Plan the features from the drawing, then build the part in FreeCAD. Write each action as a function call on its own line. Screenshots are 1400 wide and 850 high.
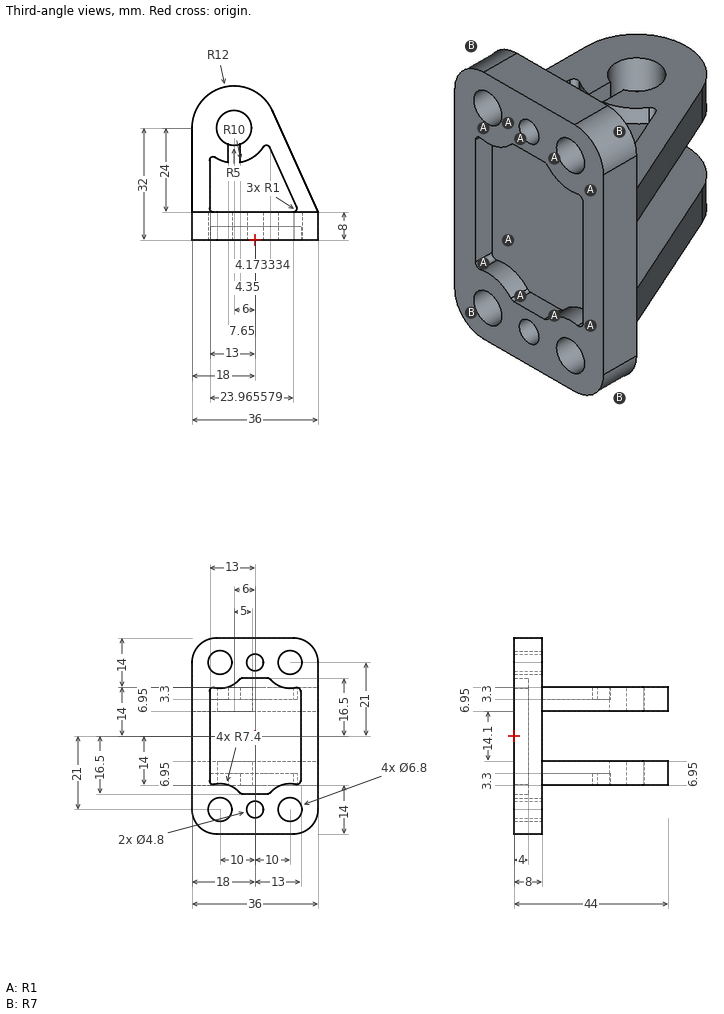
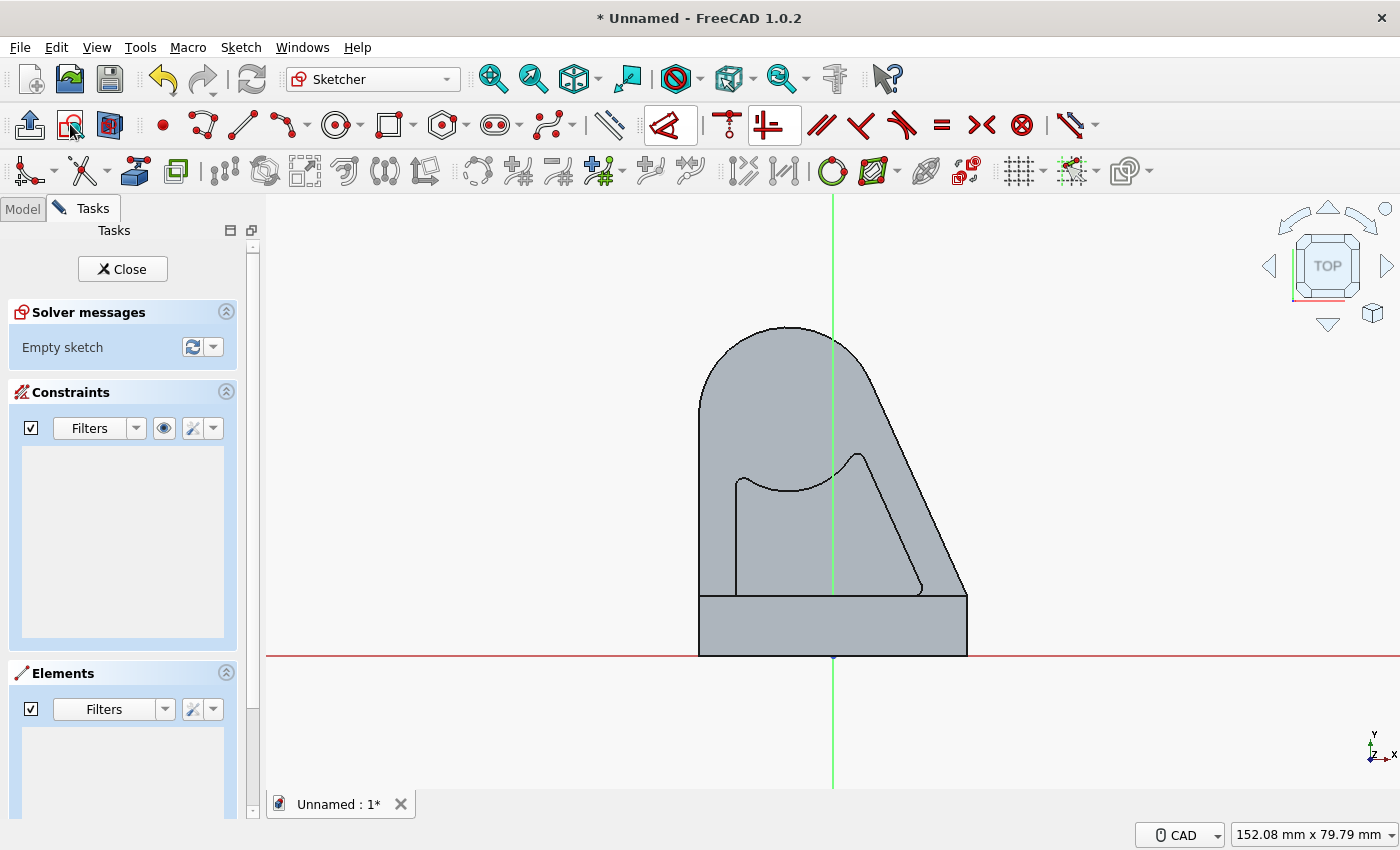
key(q)
key(s)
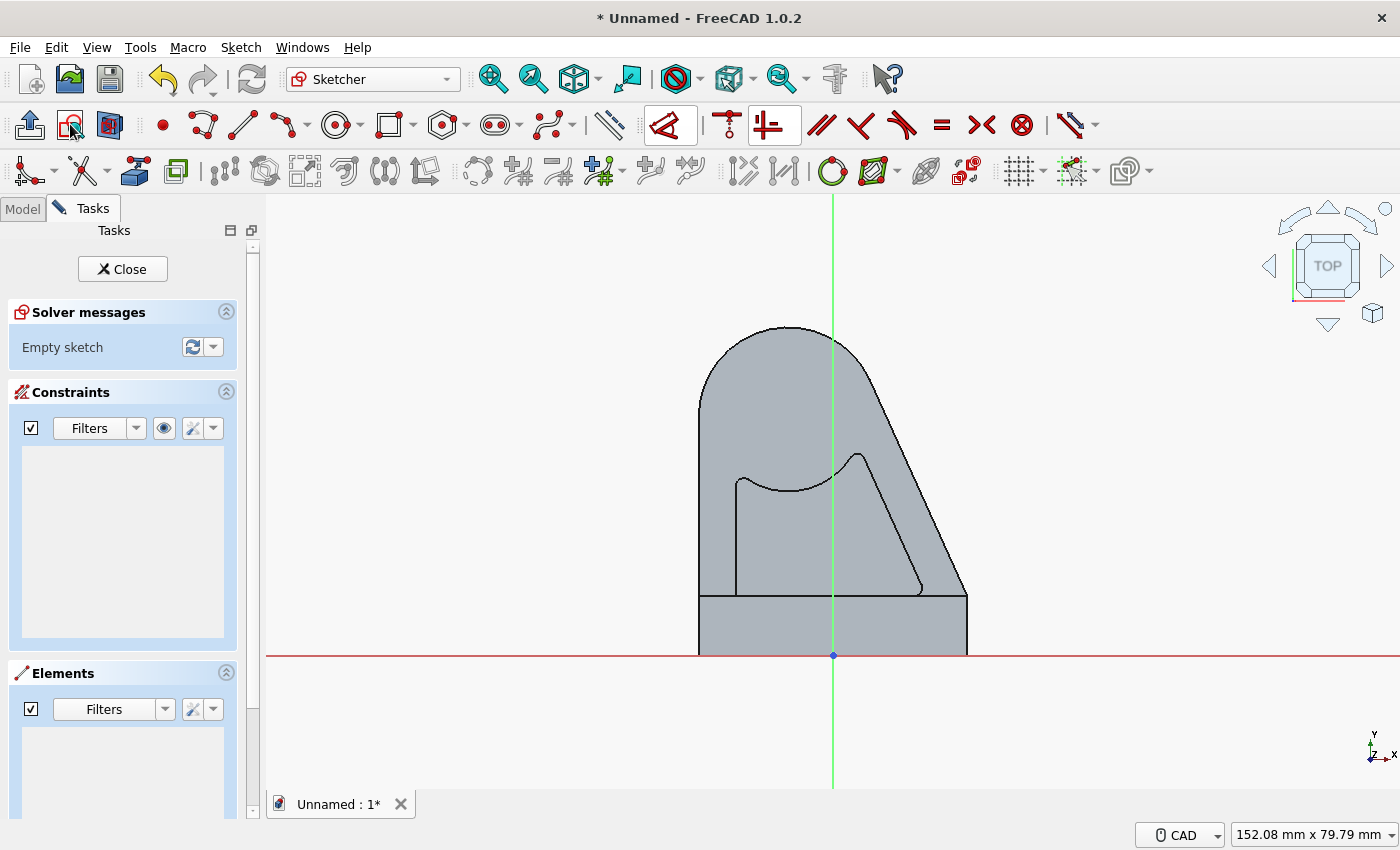
scroll(791, 469, up, 11)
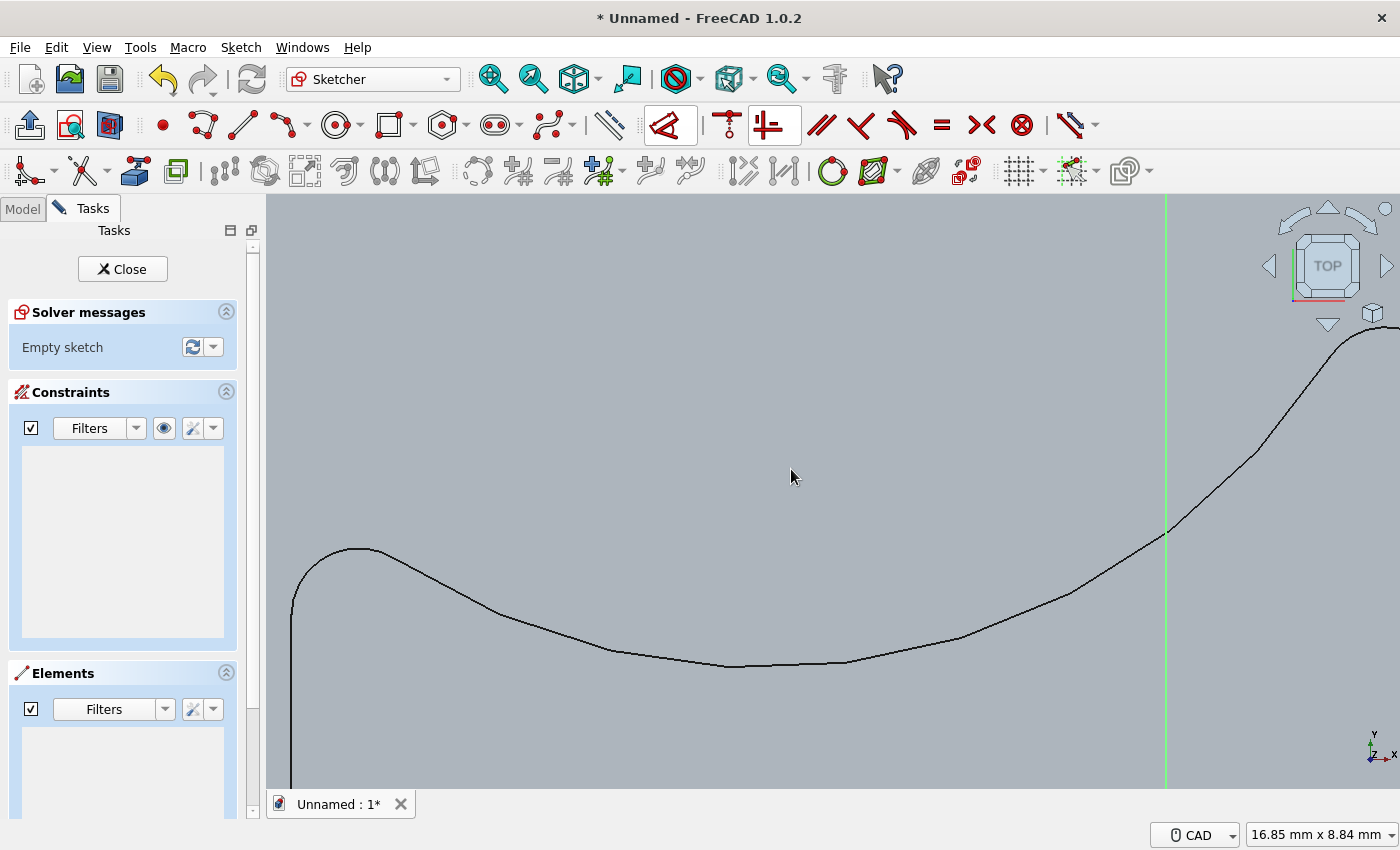
click(244, 126)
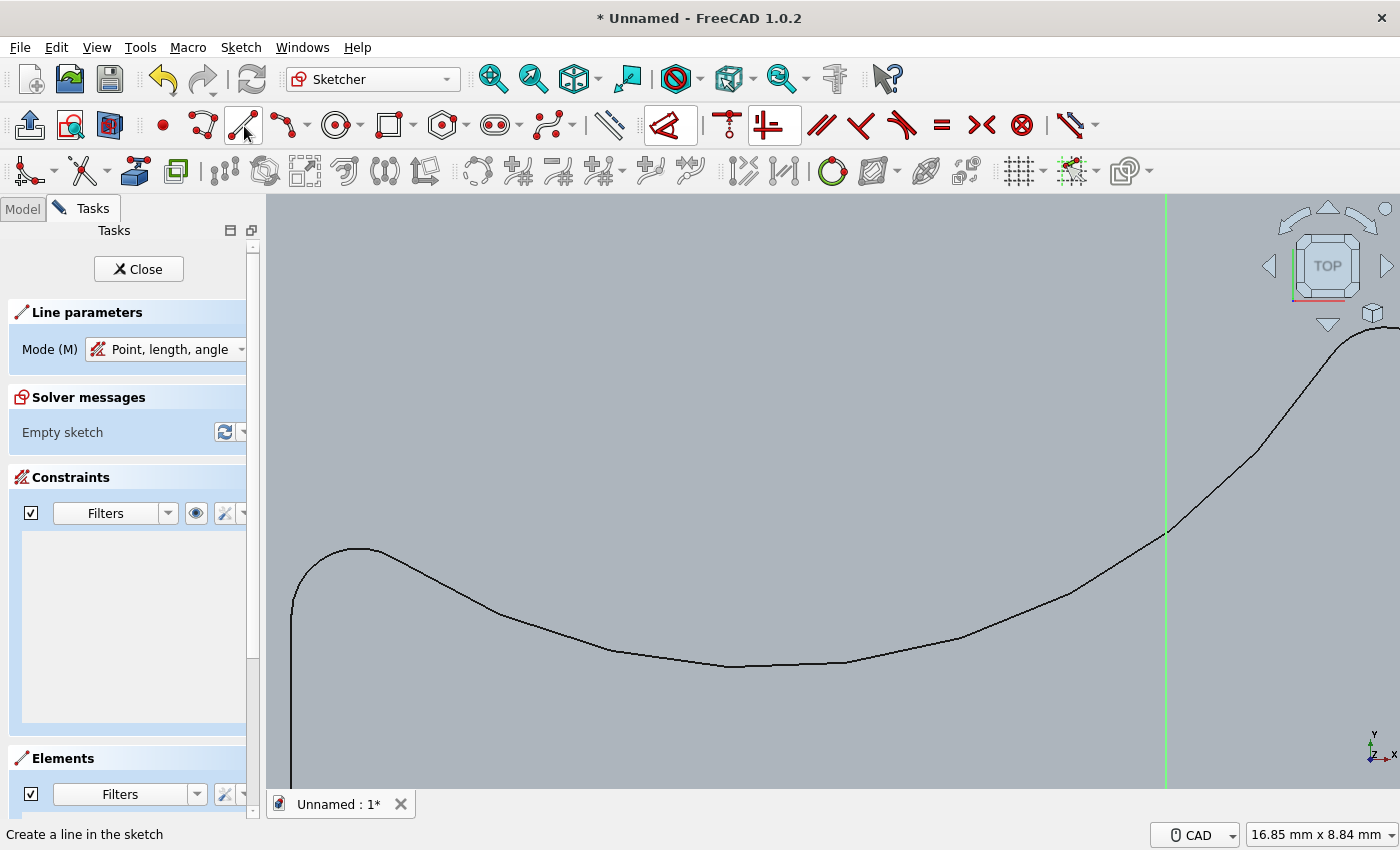
click(652, 313)
click(652, 659)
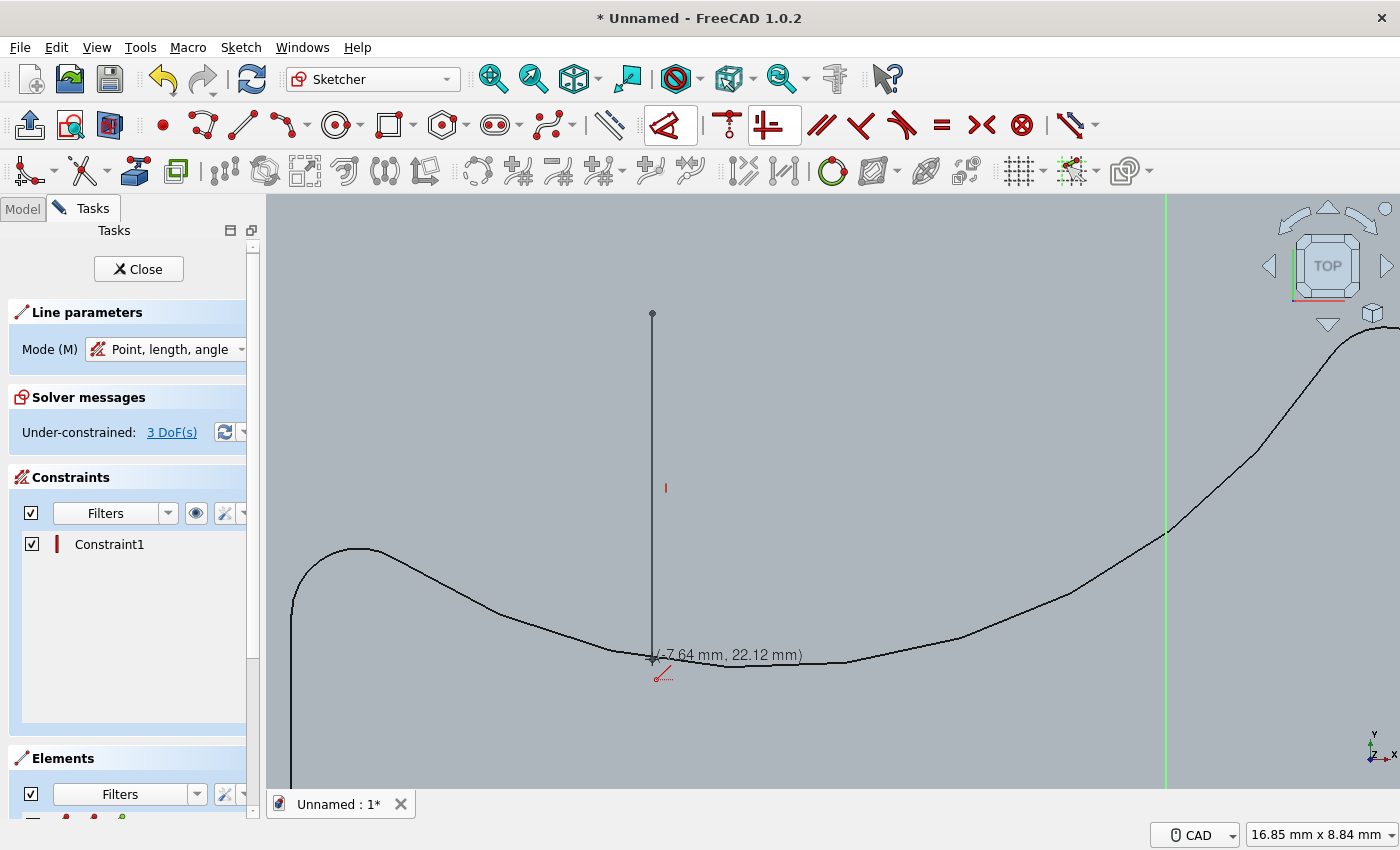
click(874, 659)
click(874, 313)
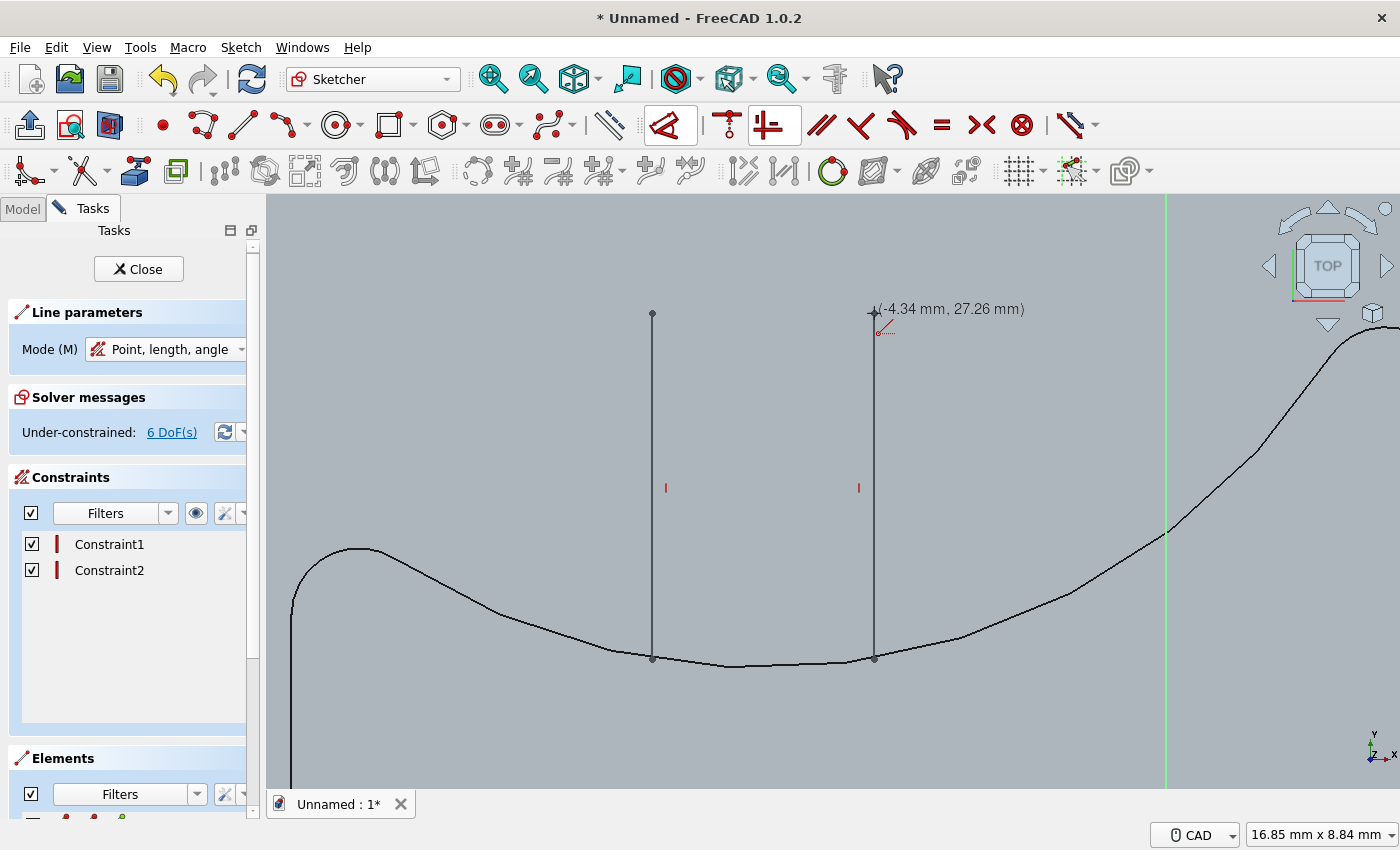
click(284, 126)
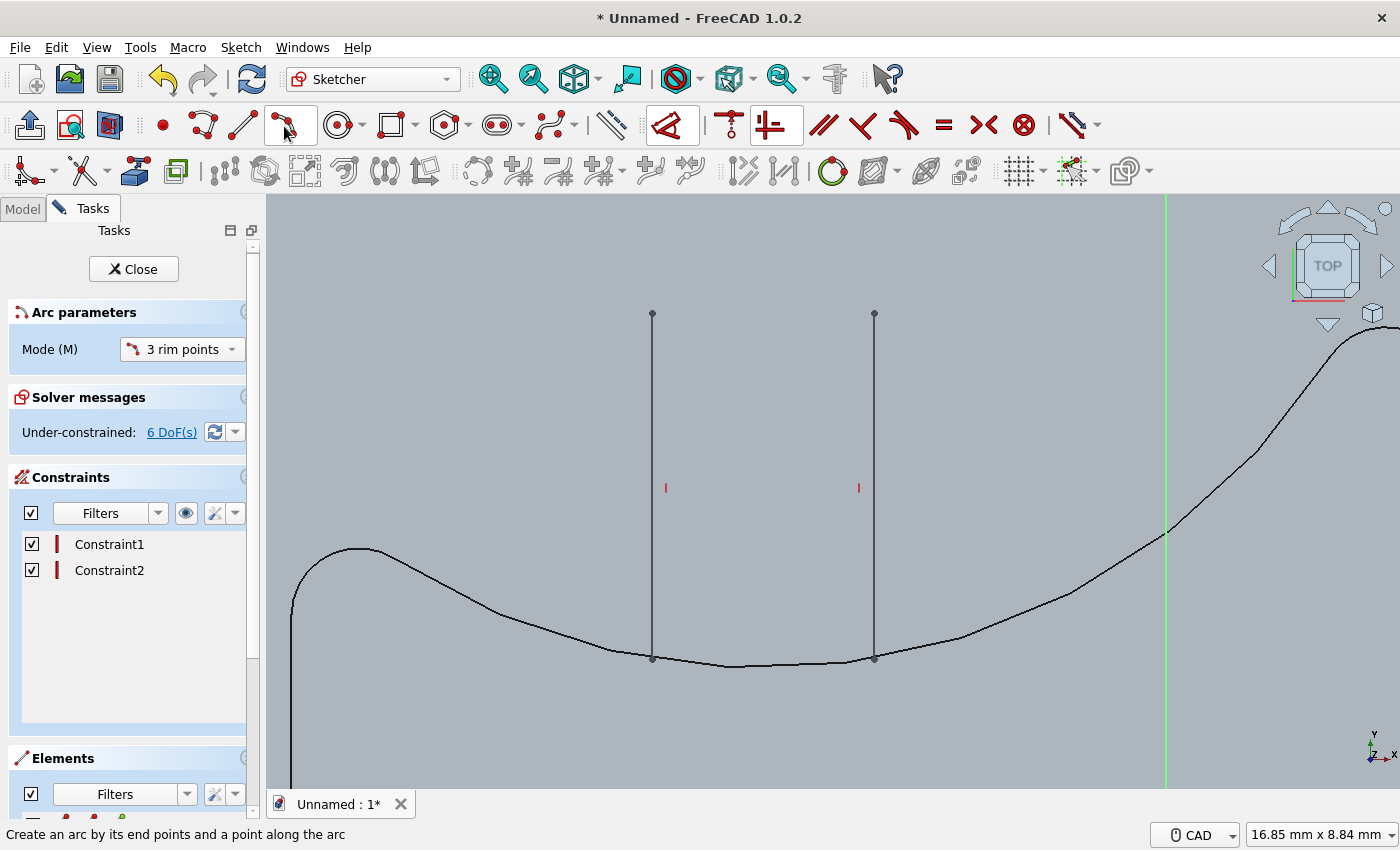
click(652, 660)
click(874, 660)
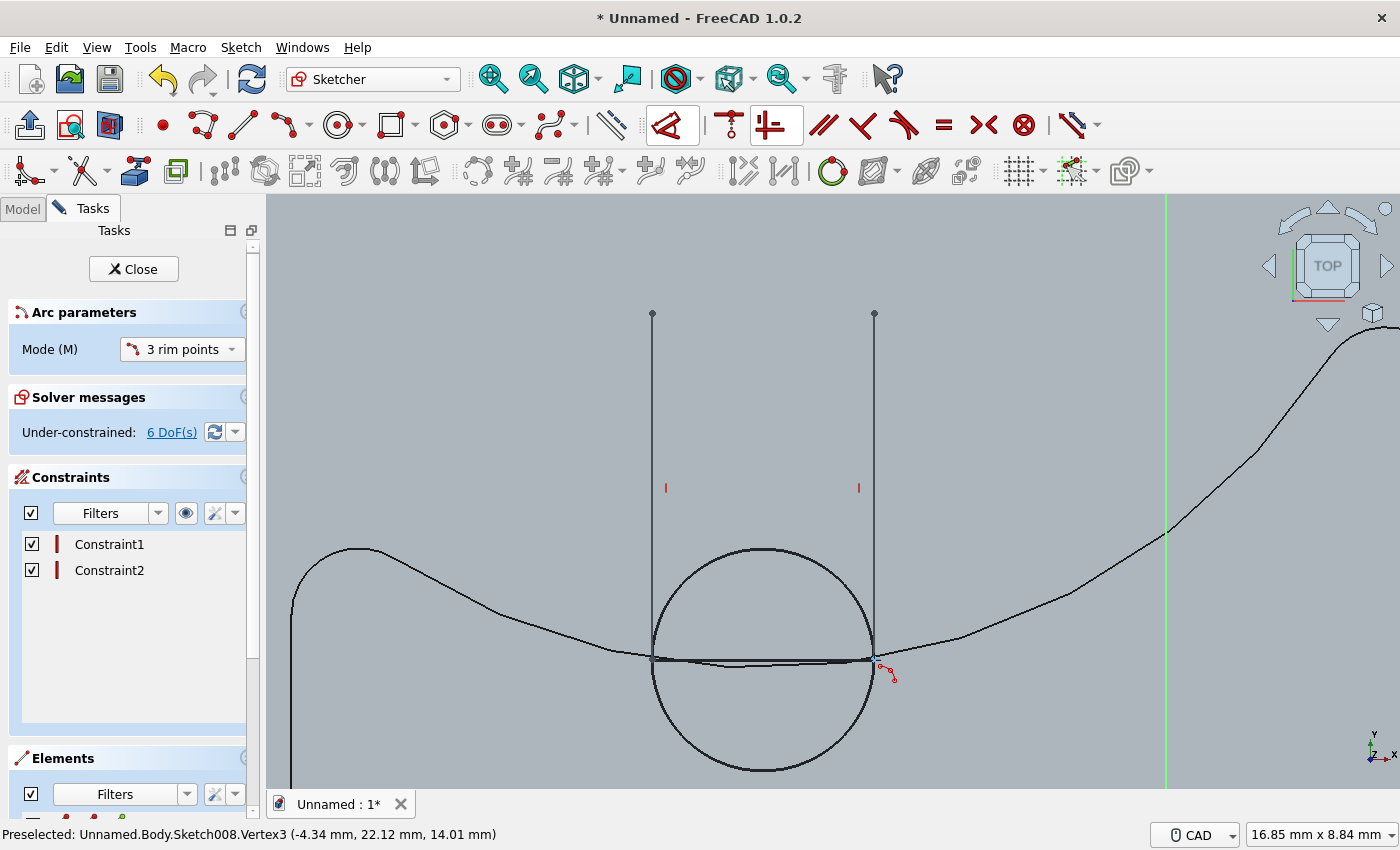
scroll(763, 668, up, 3)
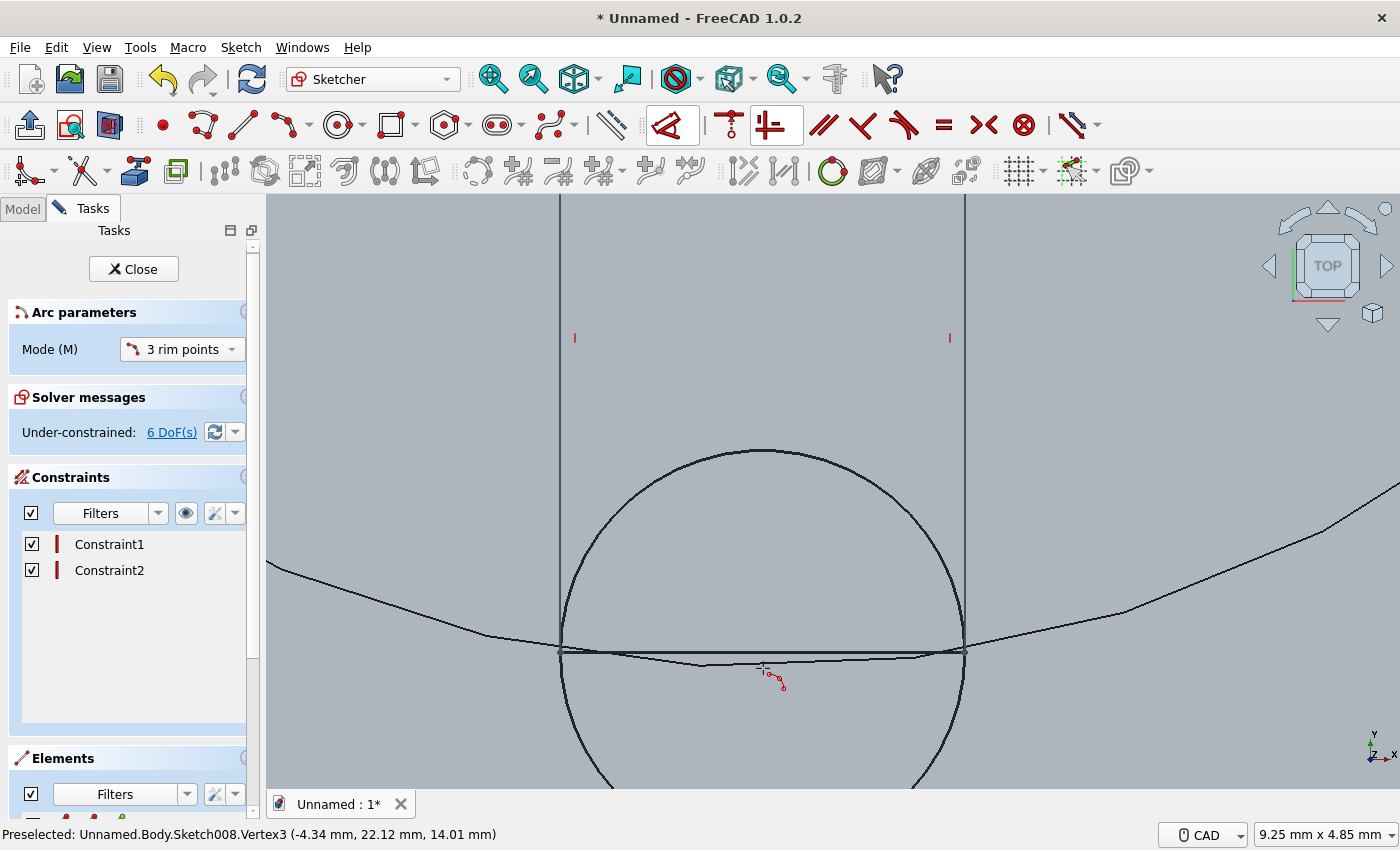
click(762, 667)